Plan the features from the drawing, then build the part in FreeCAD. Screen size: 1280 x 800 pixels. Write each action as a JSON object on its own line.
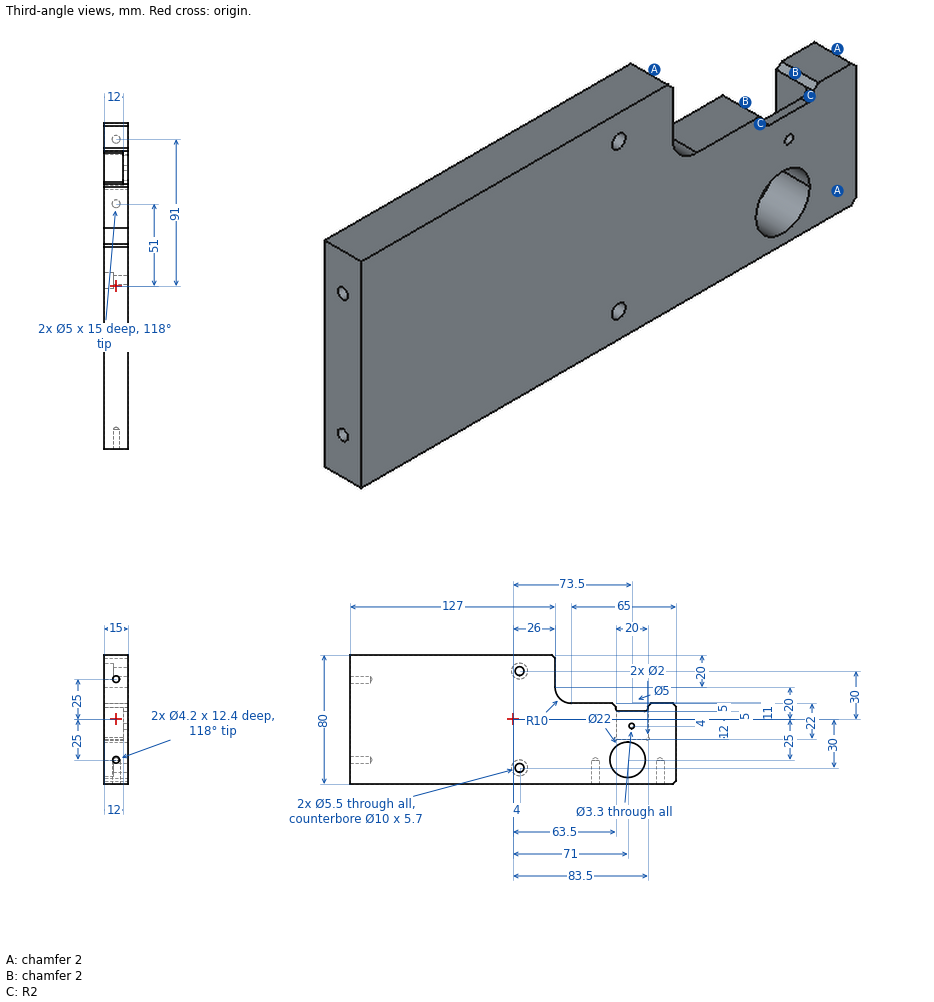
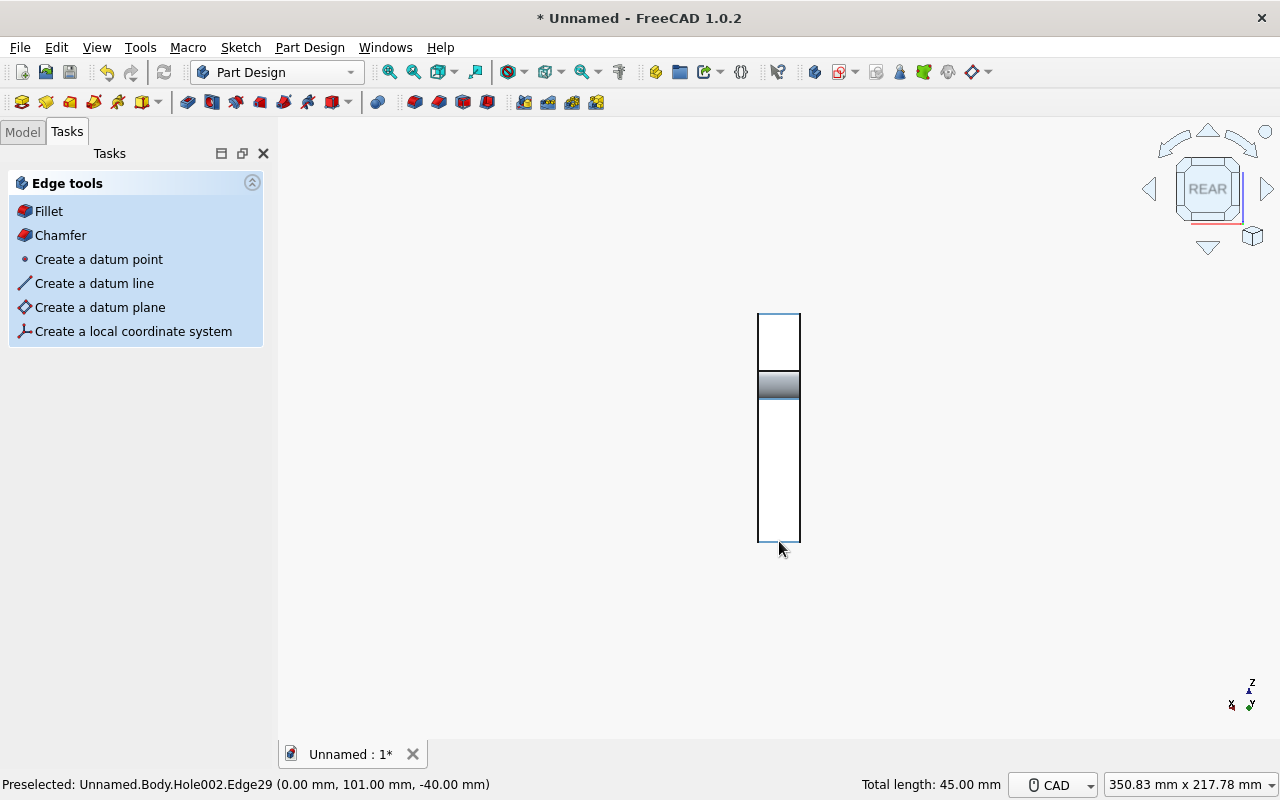
{"action": "left_click", "coordinate": [440, 102]}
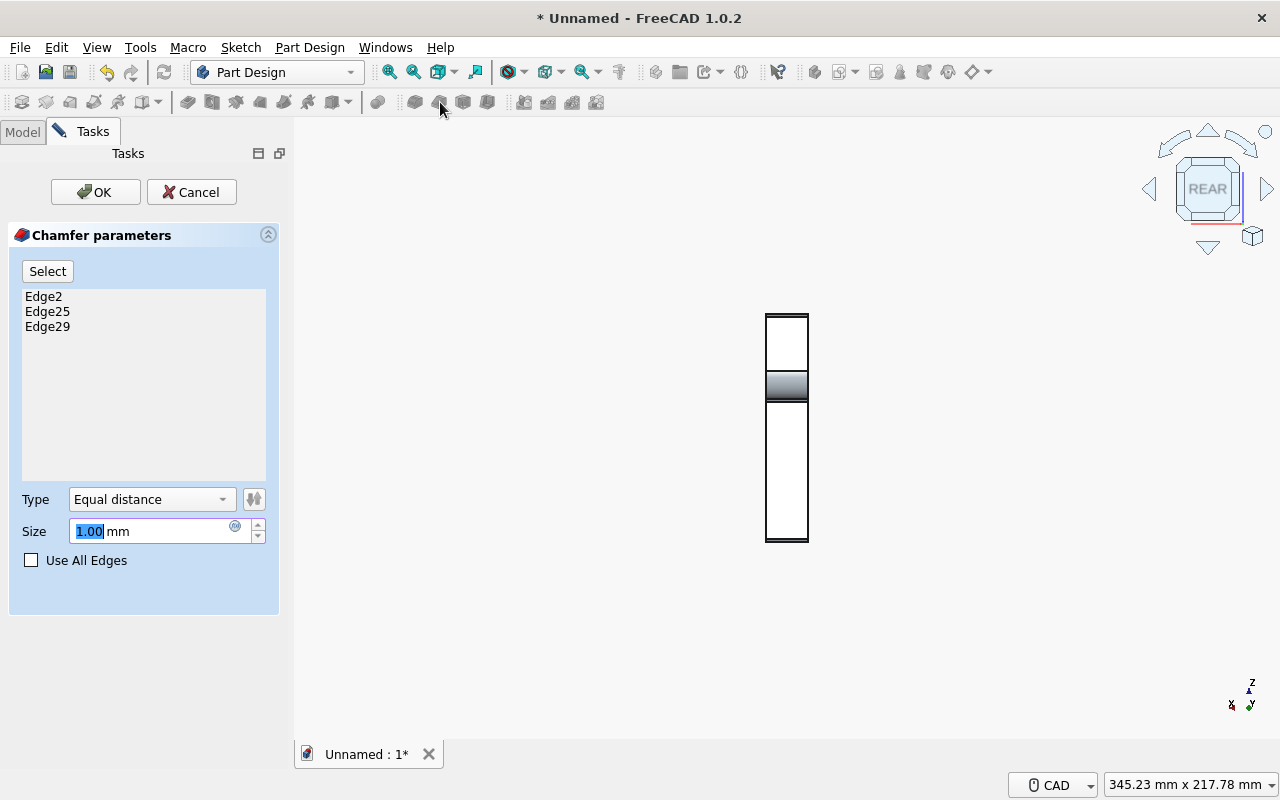
{"action": "type", "text": "2"}
{"action": "key", "text": "Tab"}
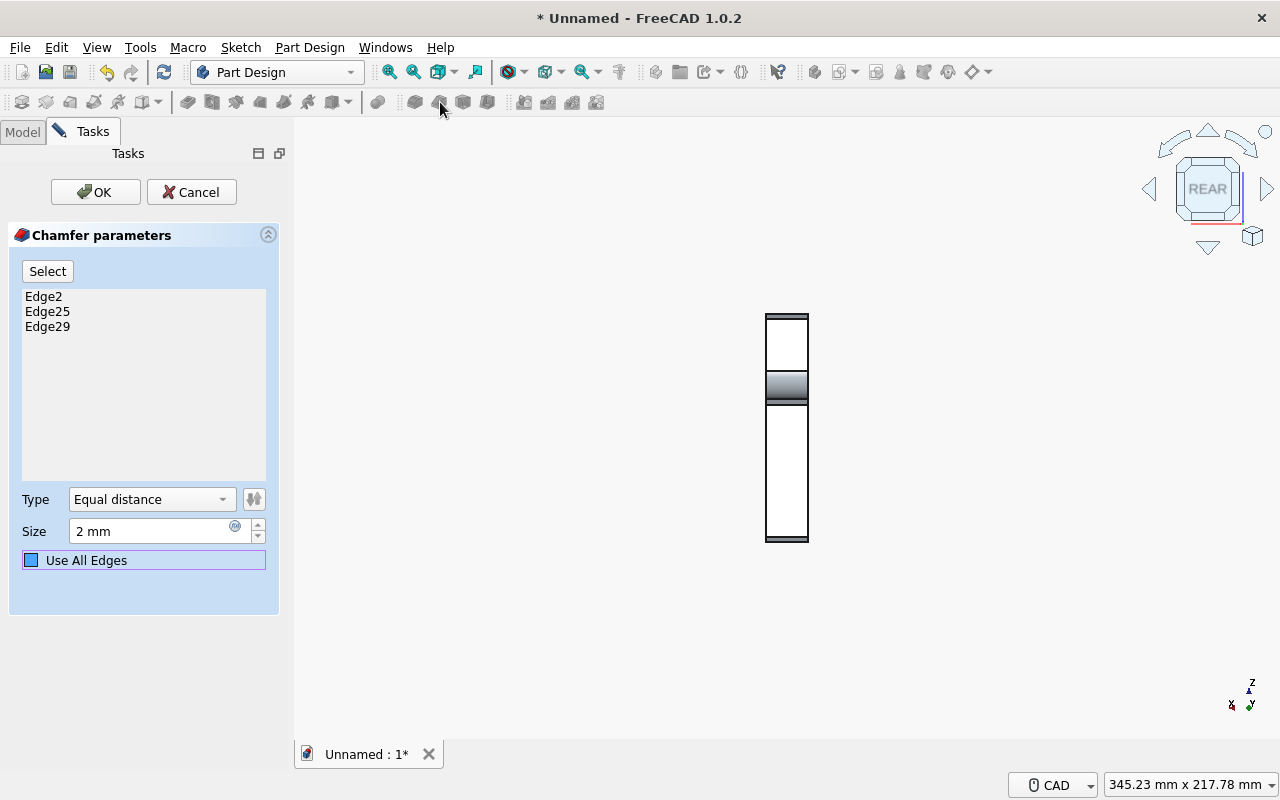
{"action": "left_click", "coordinate": [96, 192]}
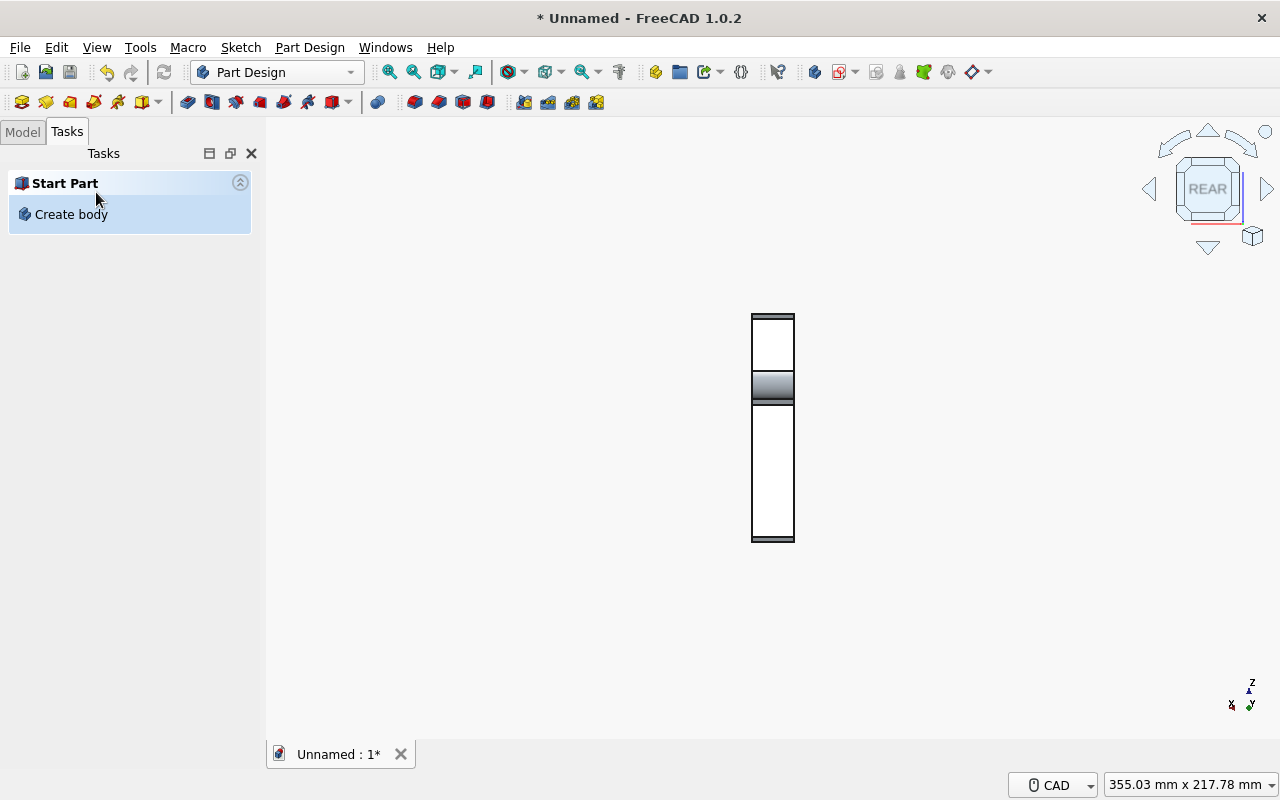
{"action": "left_click", "coordinate": [390, 72]}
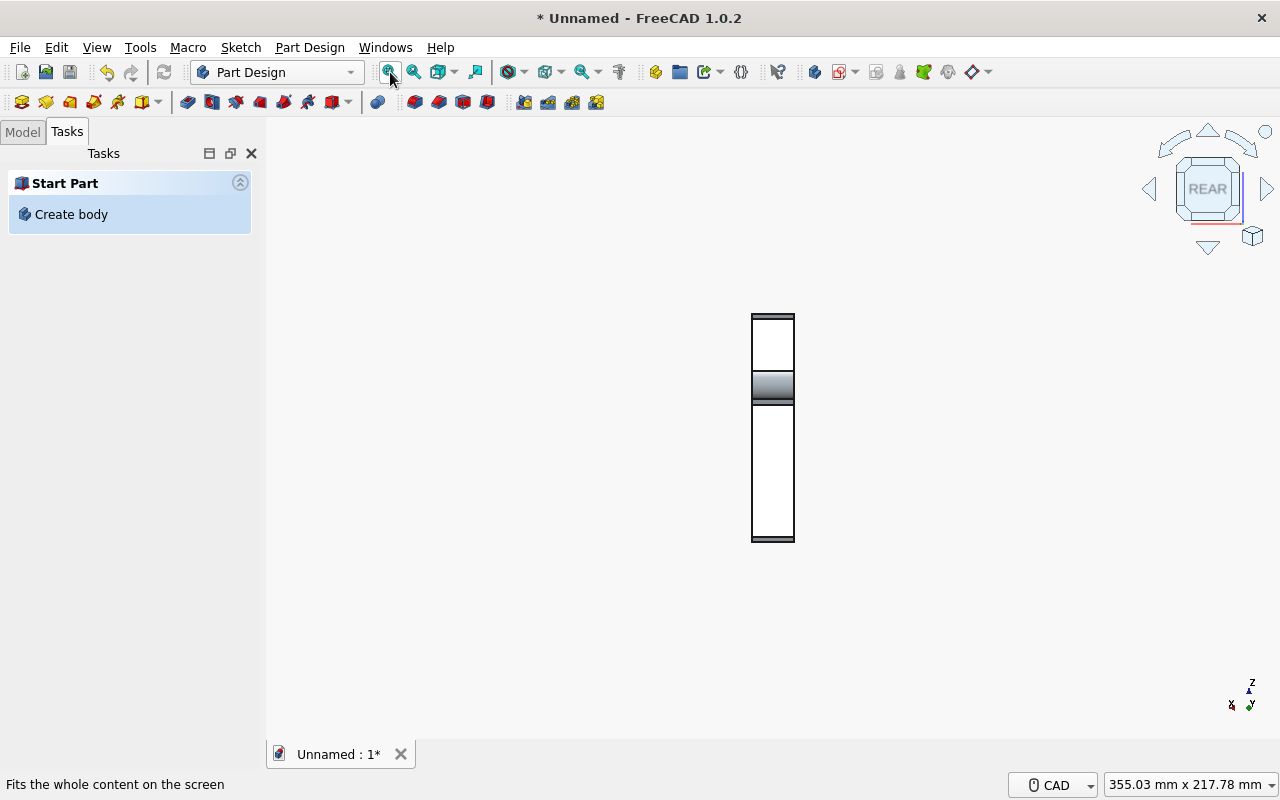
{"action": "key", "text": "0"}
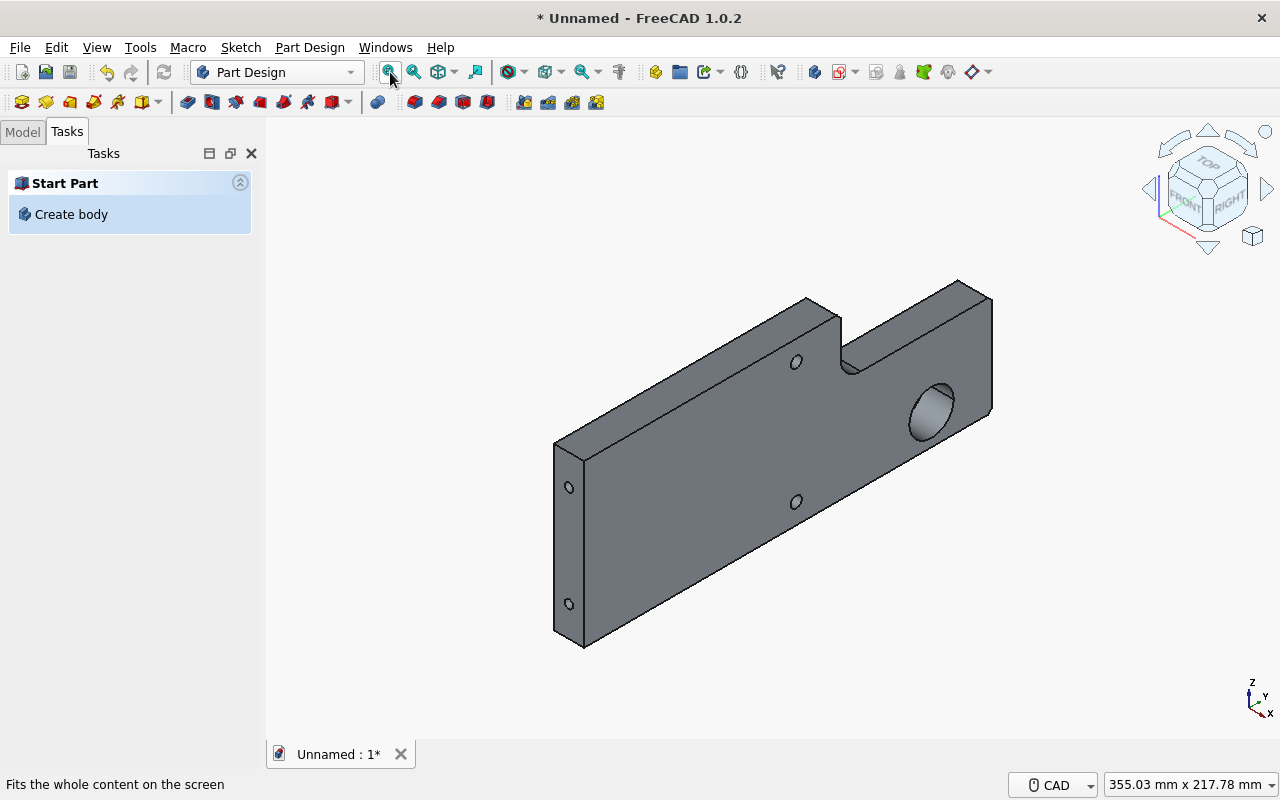
{"action": "left_click", "coordinate": [730, 469]}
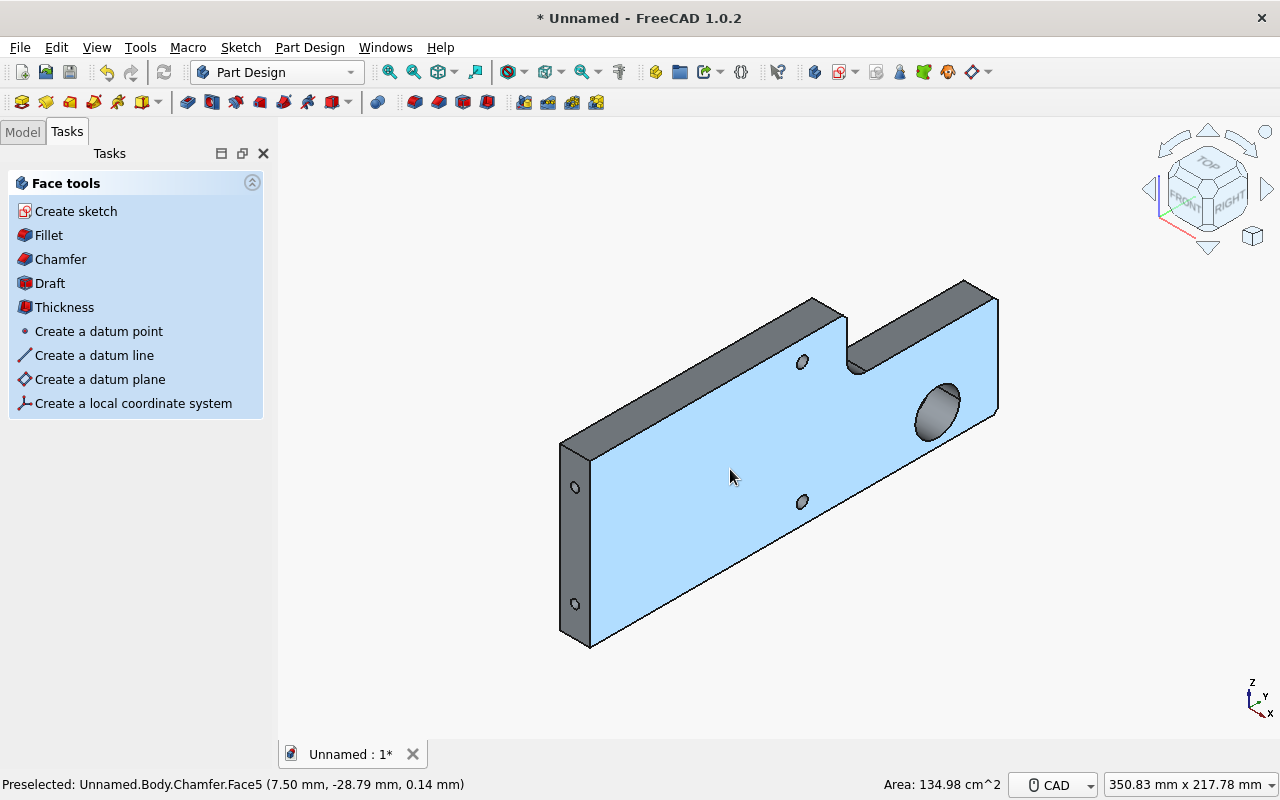
{"action": "left_click", "coordinate": [840, 72]}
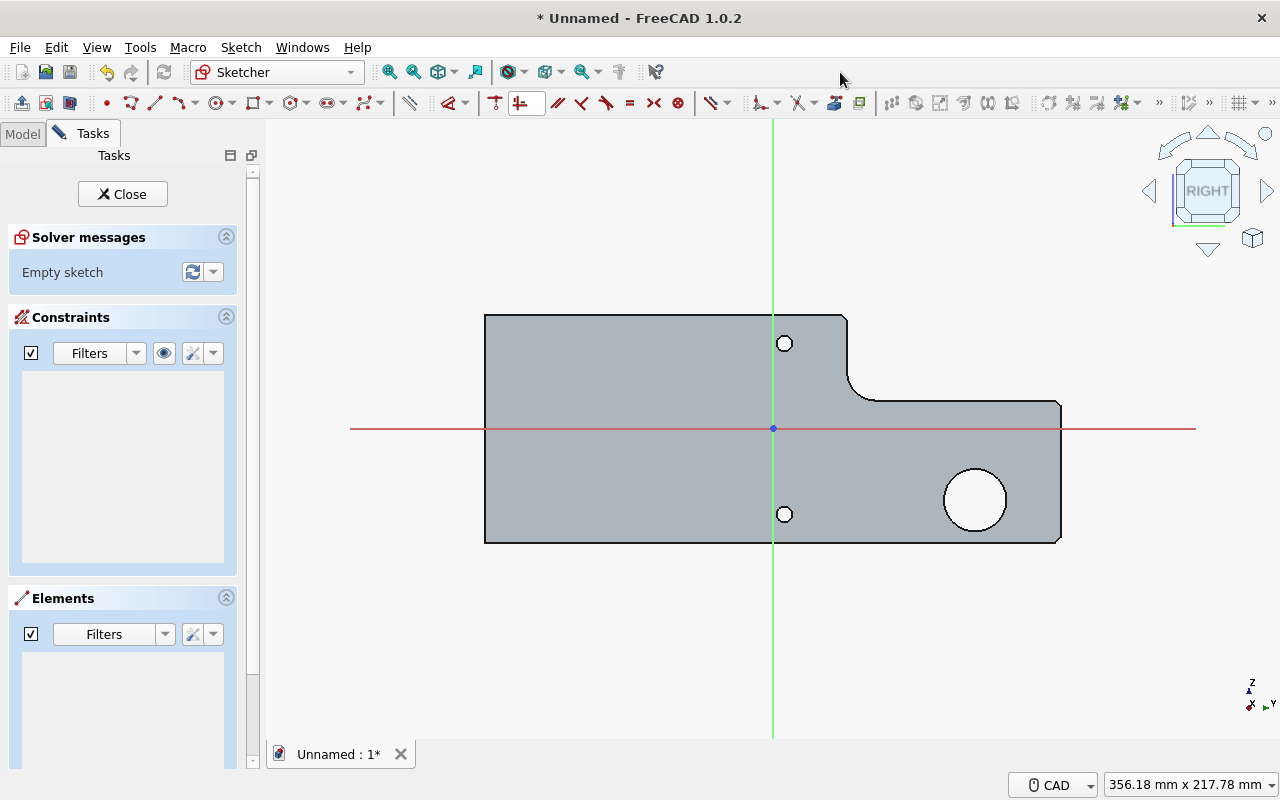
{"action": "scroll", "coordinate": [997, 396], "scroll_direction": "up", "scroll_amount": 15}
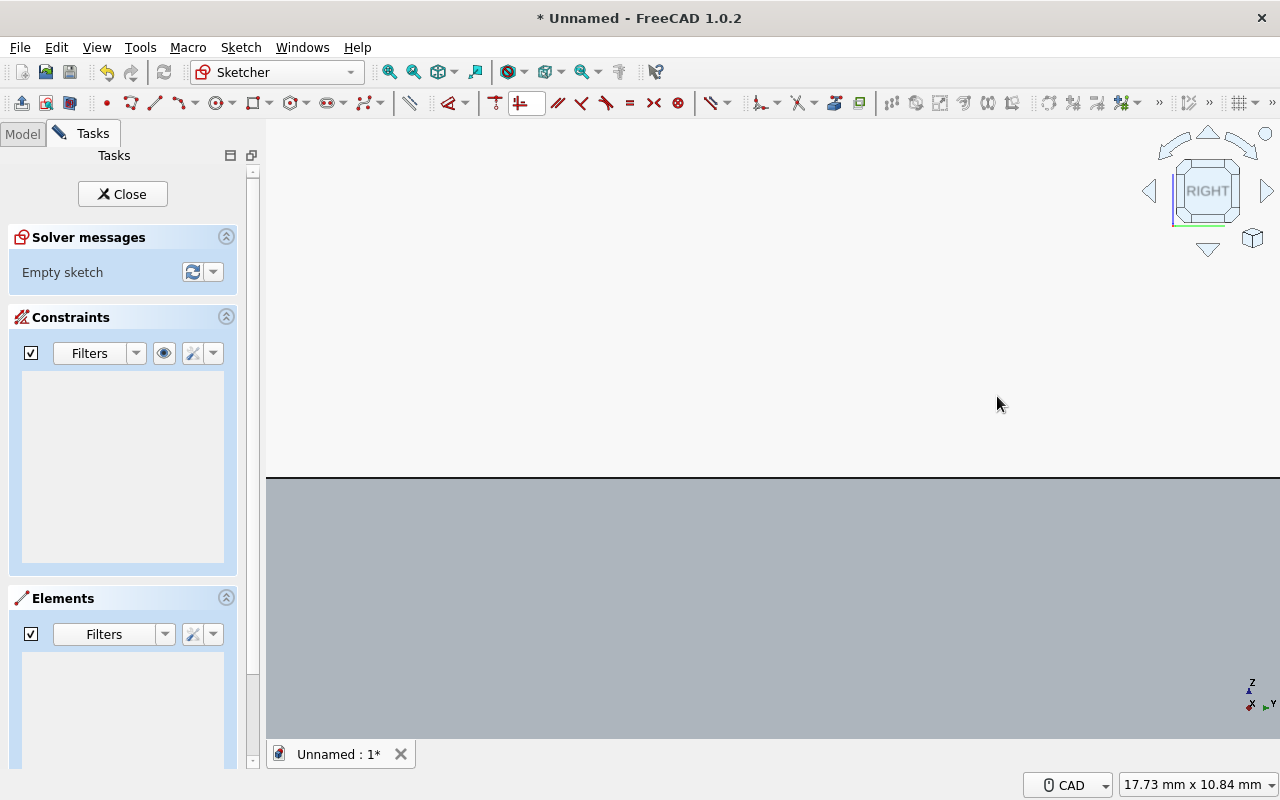
{"action": "scroll", "coordinate": [651, 406], "scroll_direction": "up", "scroll_amount": 2}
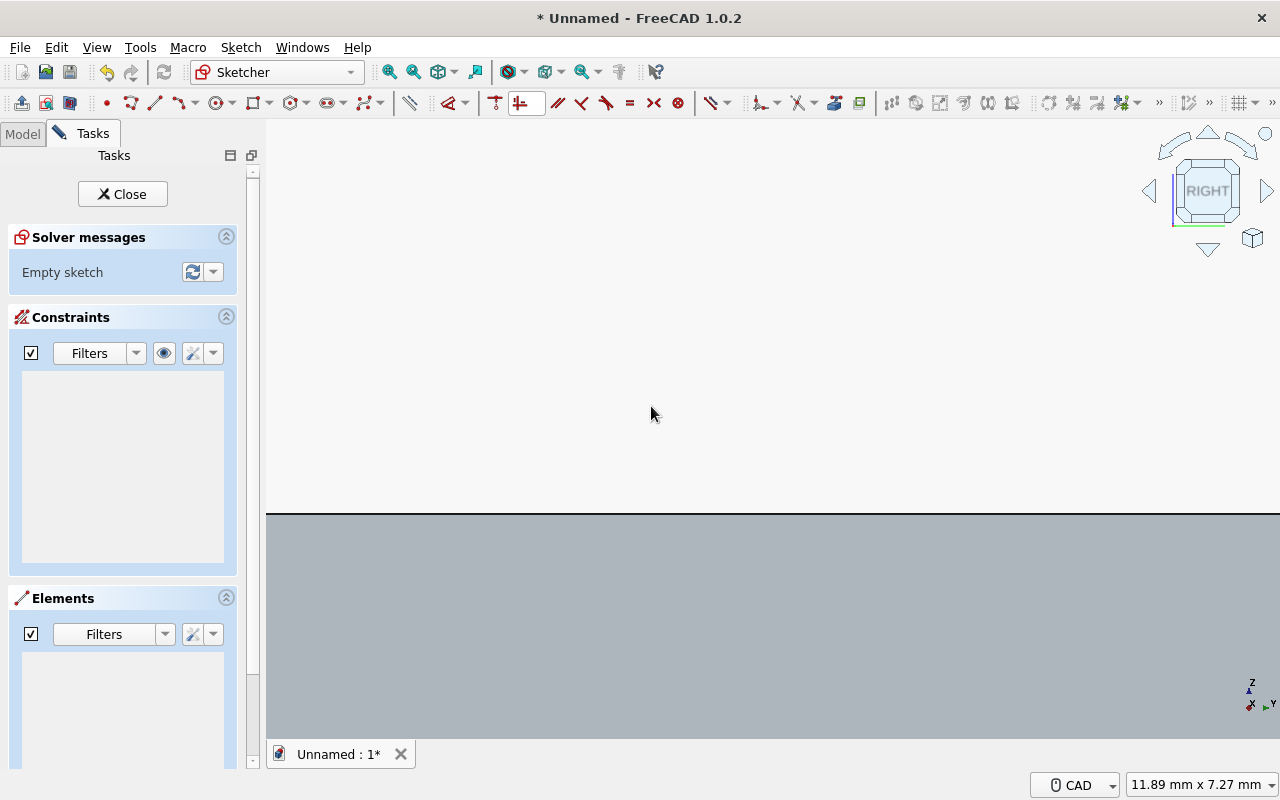
{"action": "left_click", "coordinate": [216, 104]}